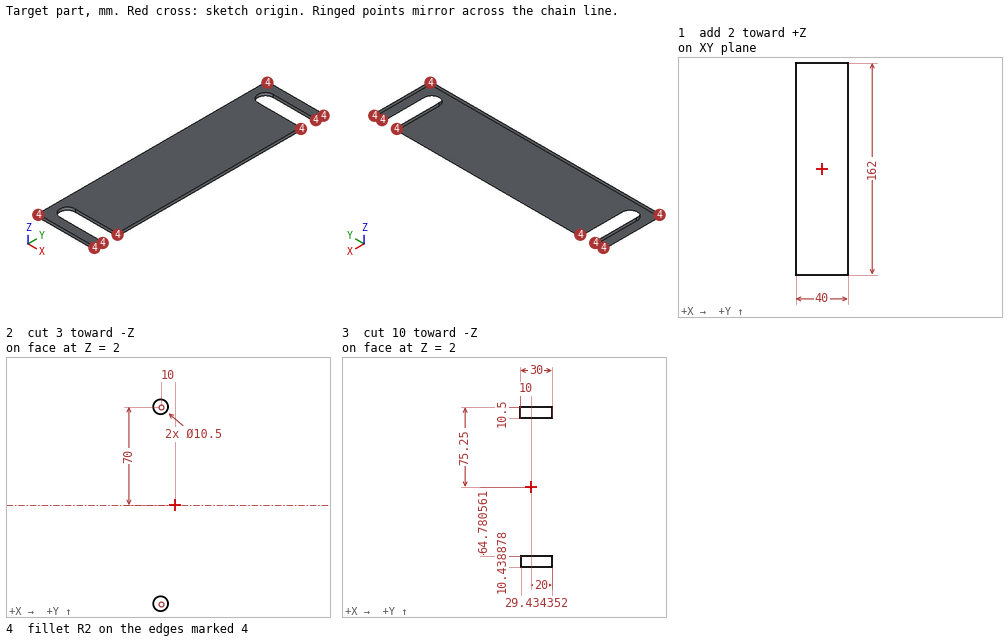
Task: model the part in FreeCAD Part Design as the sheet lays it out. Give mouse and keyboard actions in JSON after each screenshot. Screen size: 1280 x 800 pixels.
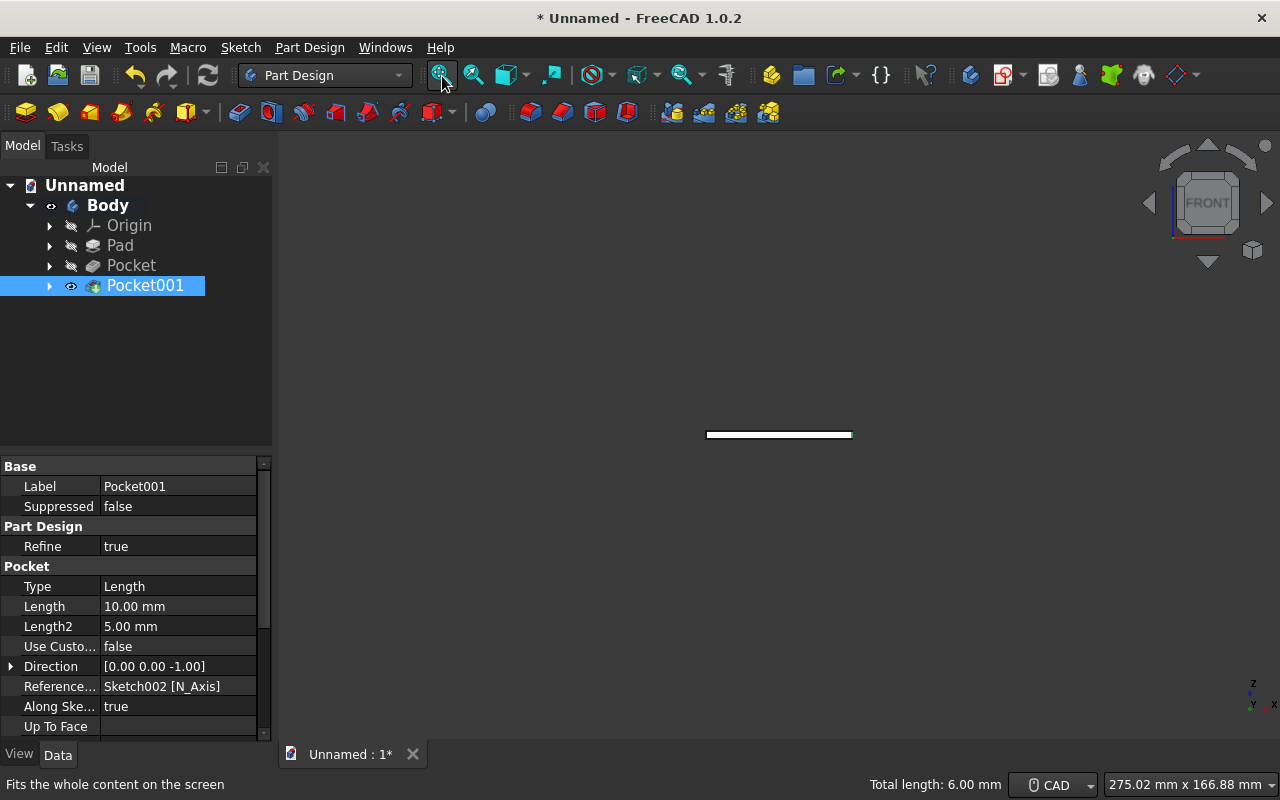
{"action": "left_click", "coordinate": [442, 76]}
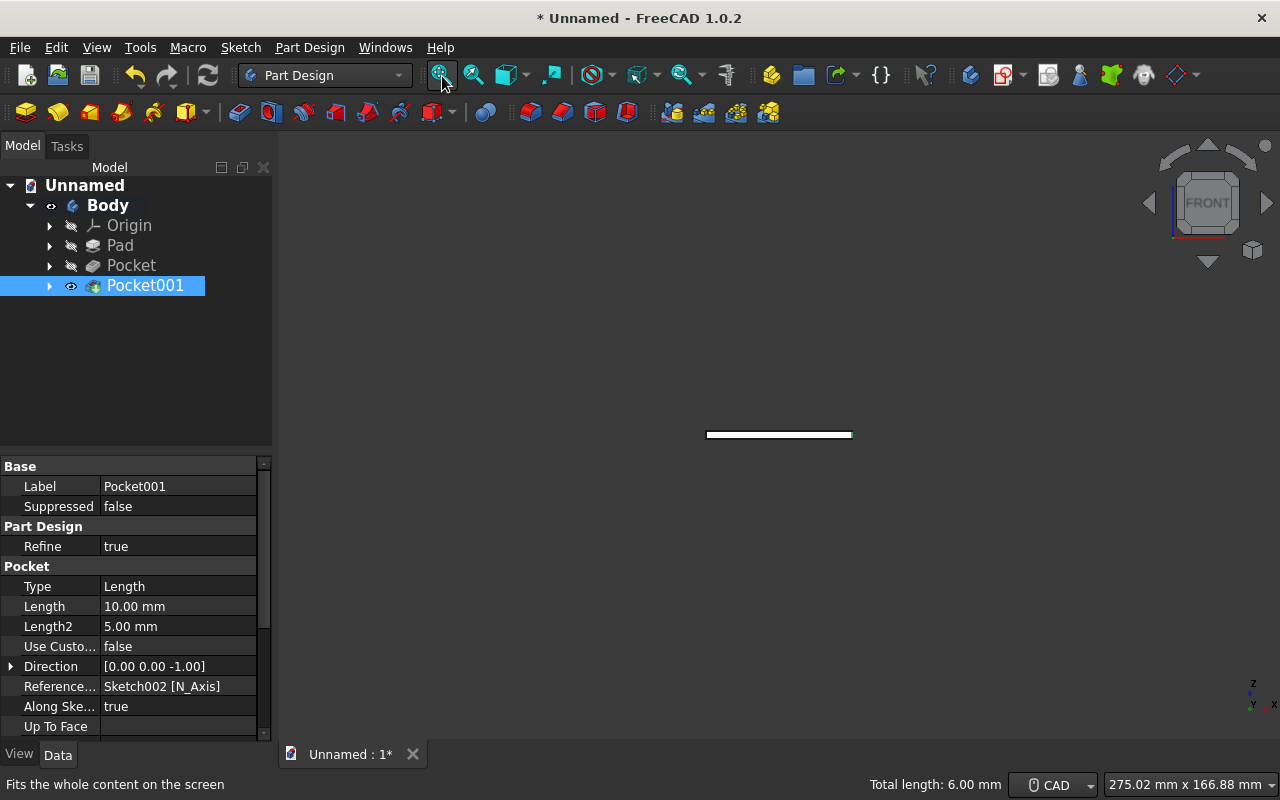
{"action": "scroll", "coordinate": [852, 434], "scroll_direction": "up", "scroll_amount": 9}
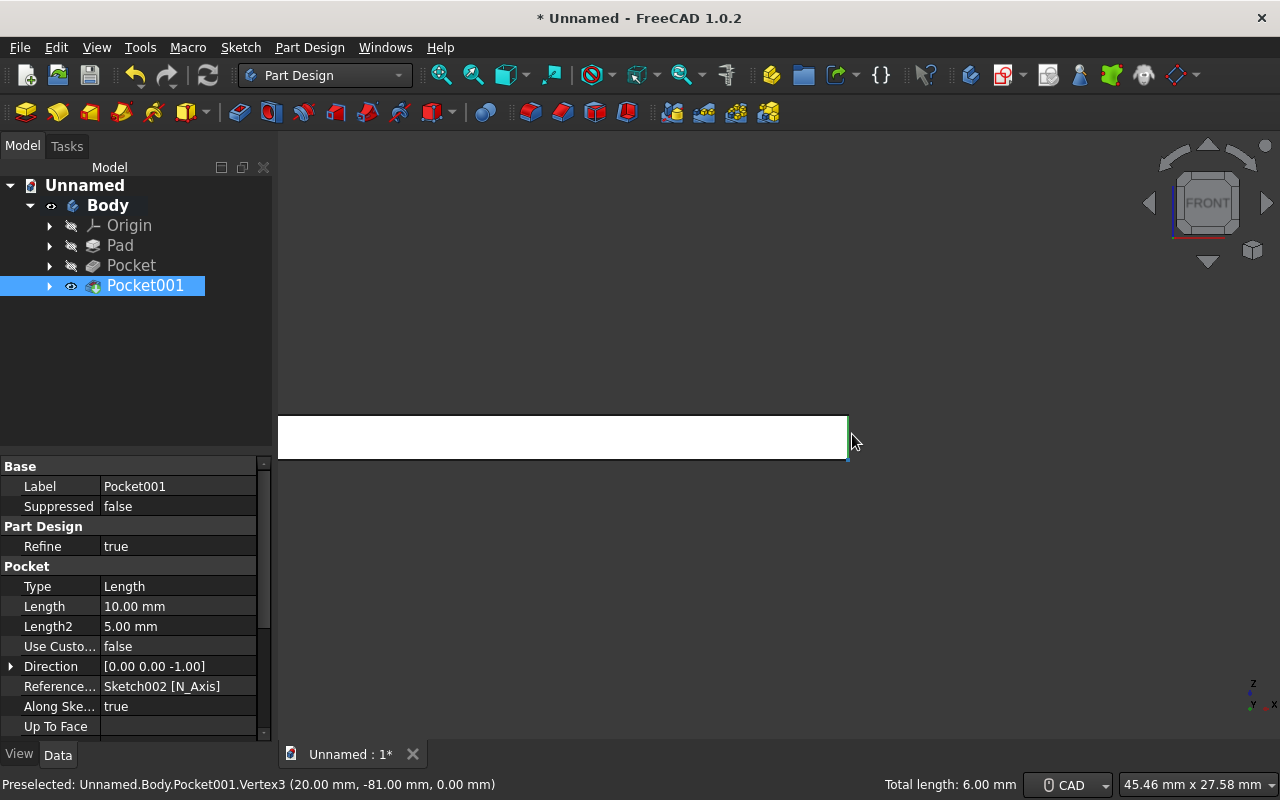
{"action": "left_click", "coordinate": [442, 76]}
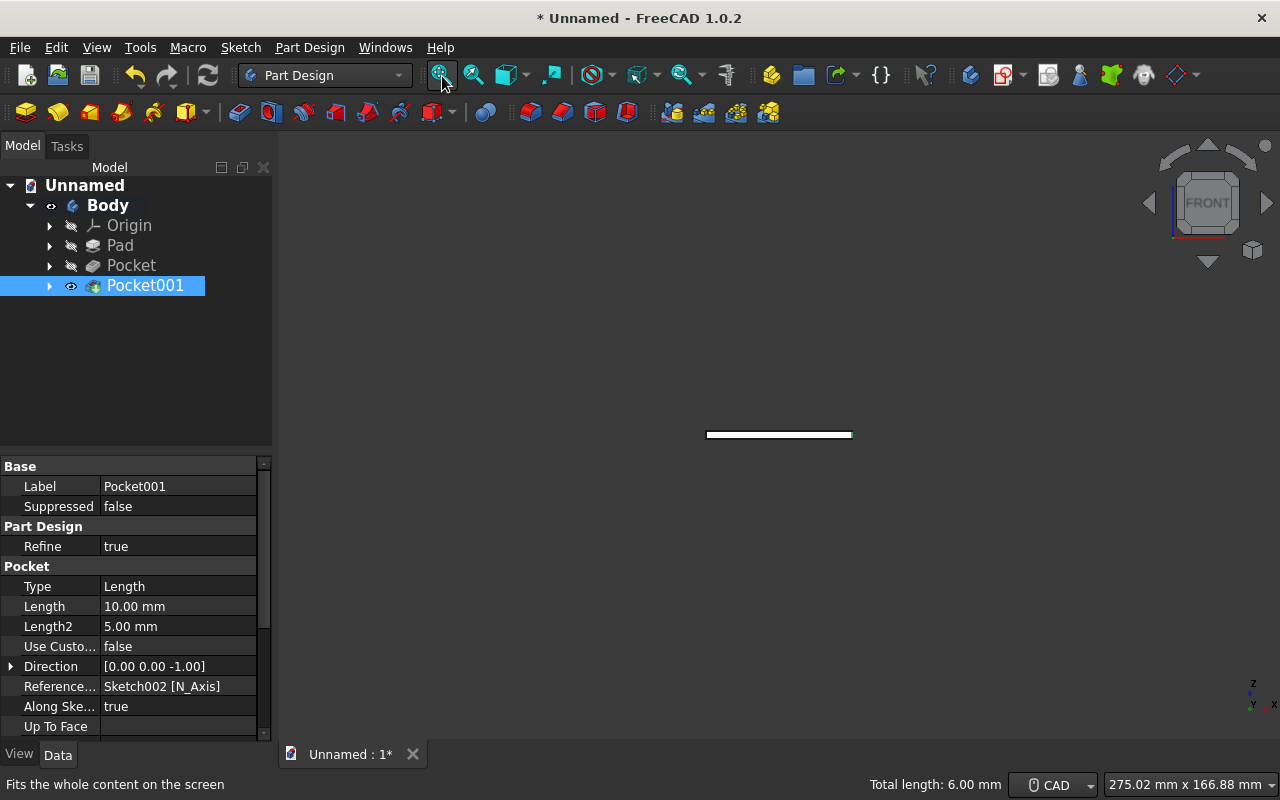
{"action": "key", "text": "3"}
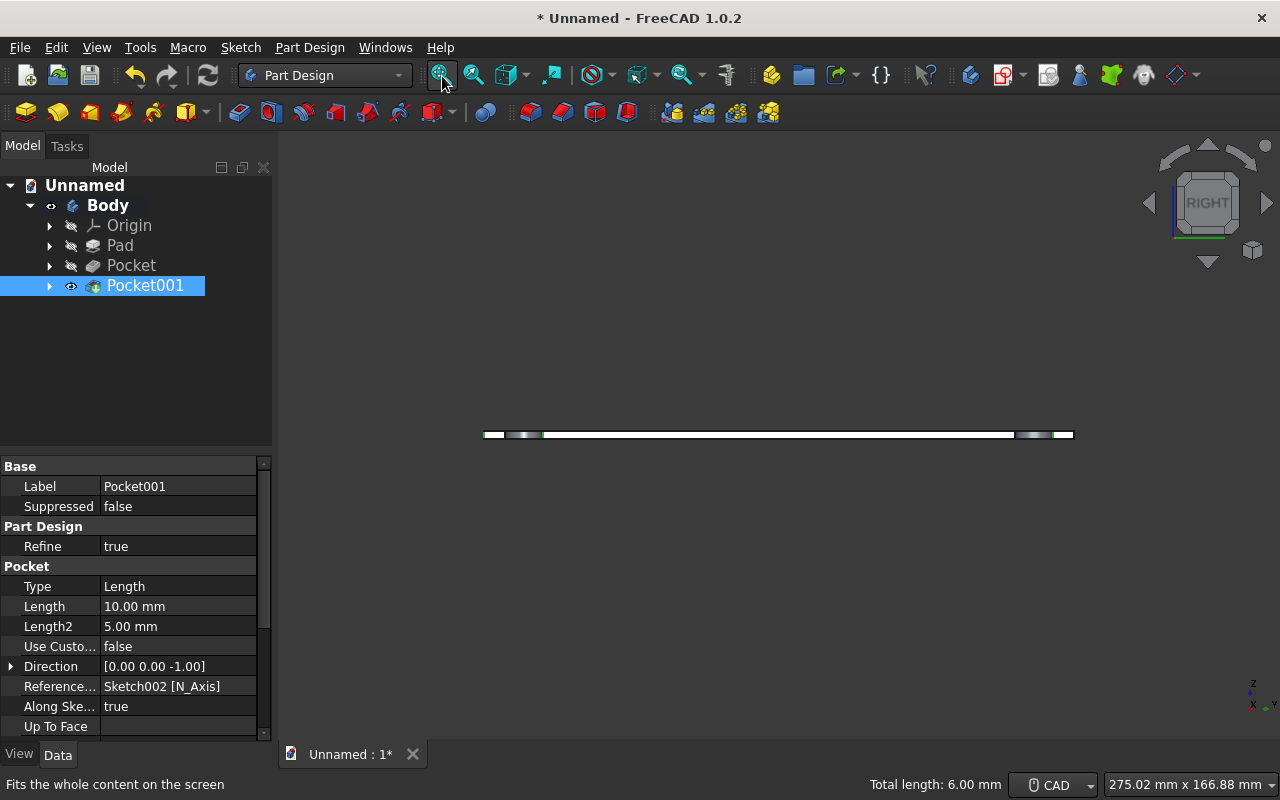
{"action": "scroll", "coordinate": [1015, 434], "scroll_direction": "up", "scroll_amount": 9}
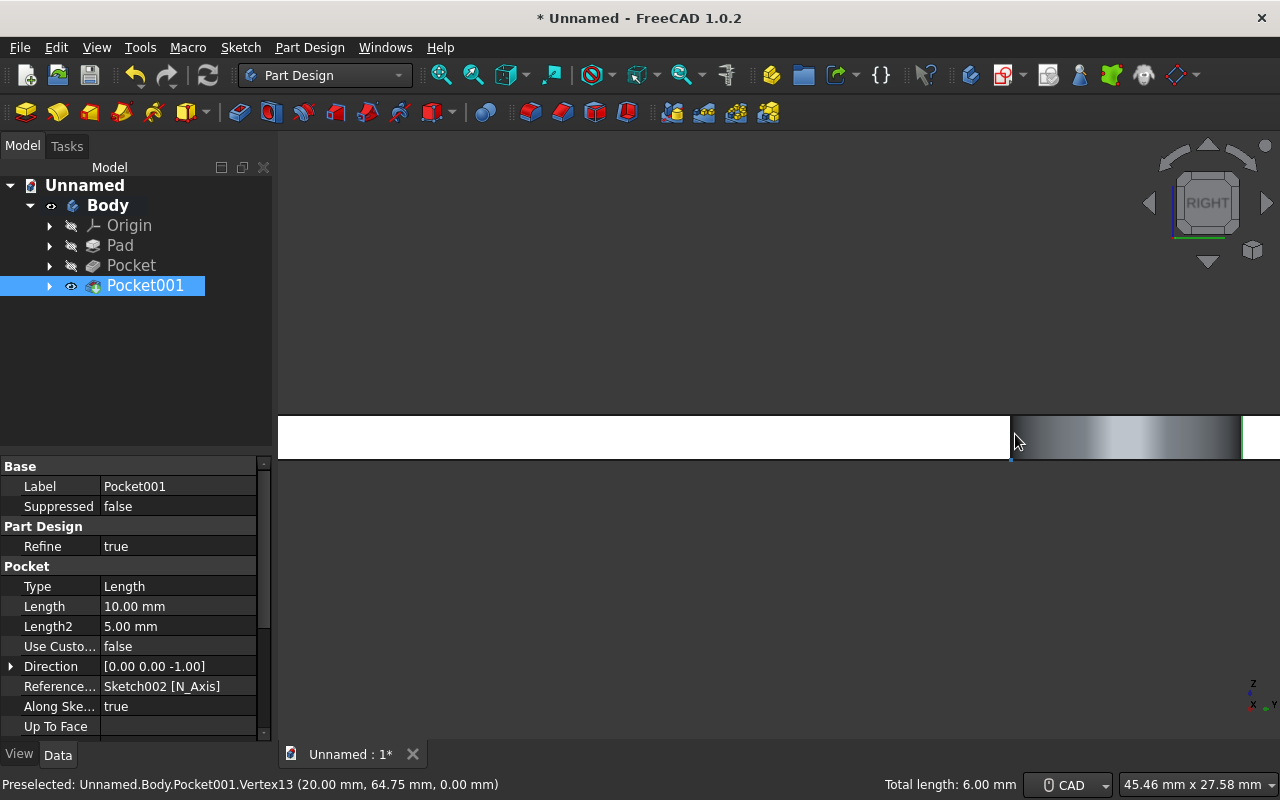
{"action": "left_click", "coordinate": [1011, 437], "text": "ctrl"}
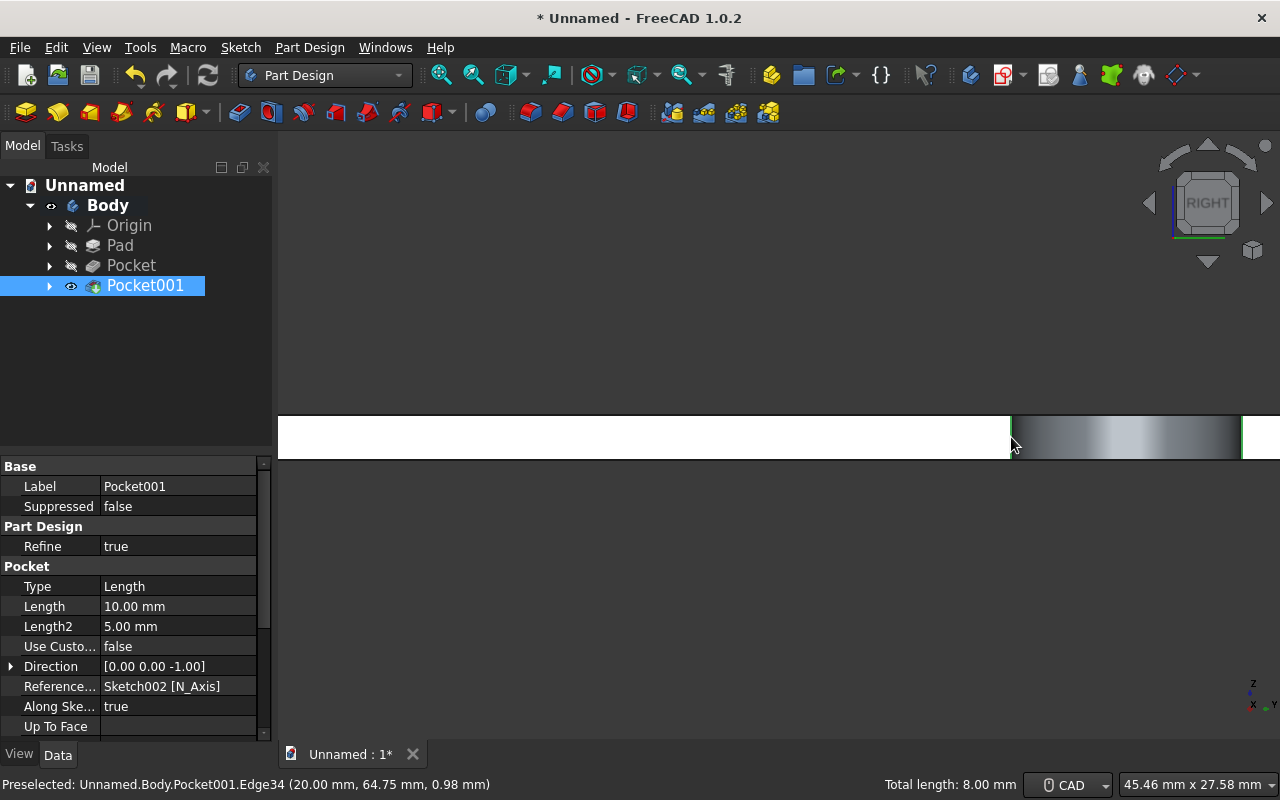
{"action": "key", "text": "v f"}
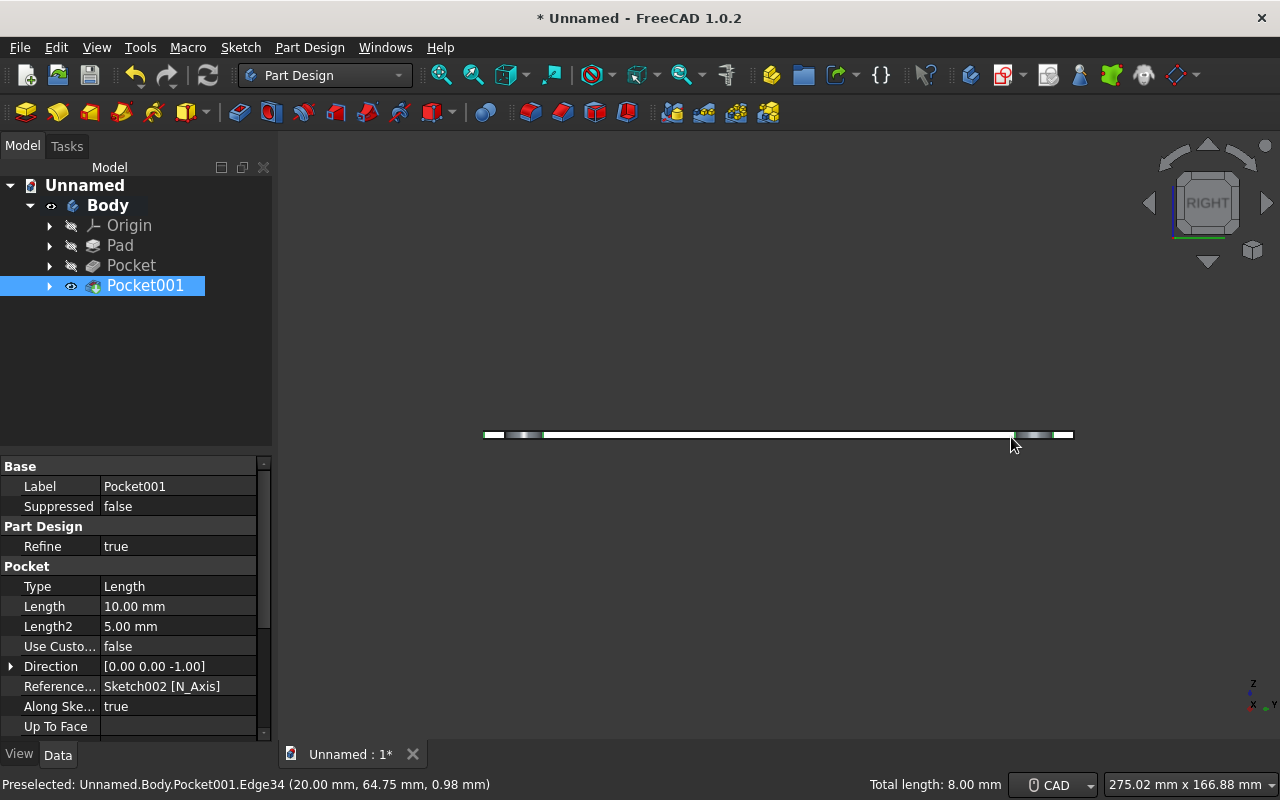
{"action": "key", "text": "5"}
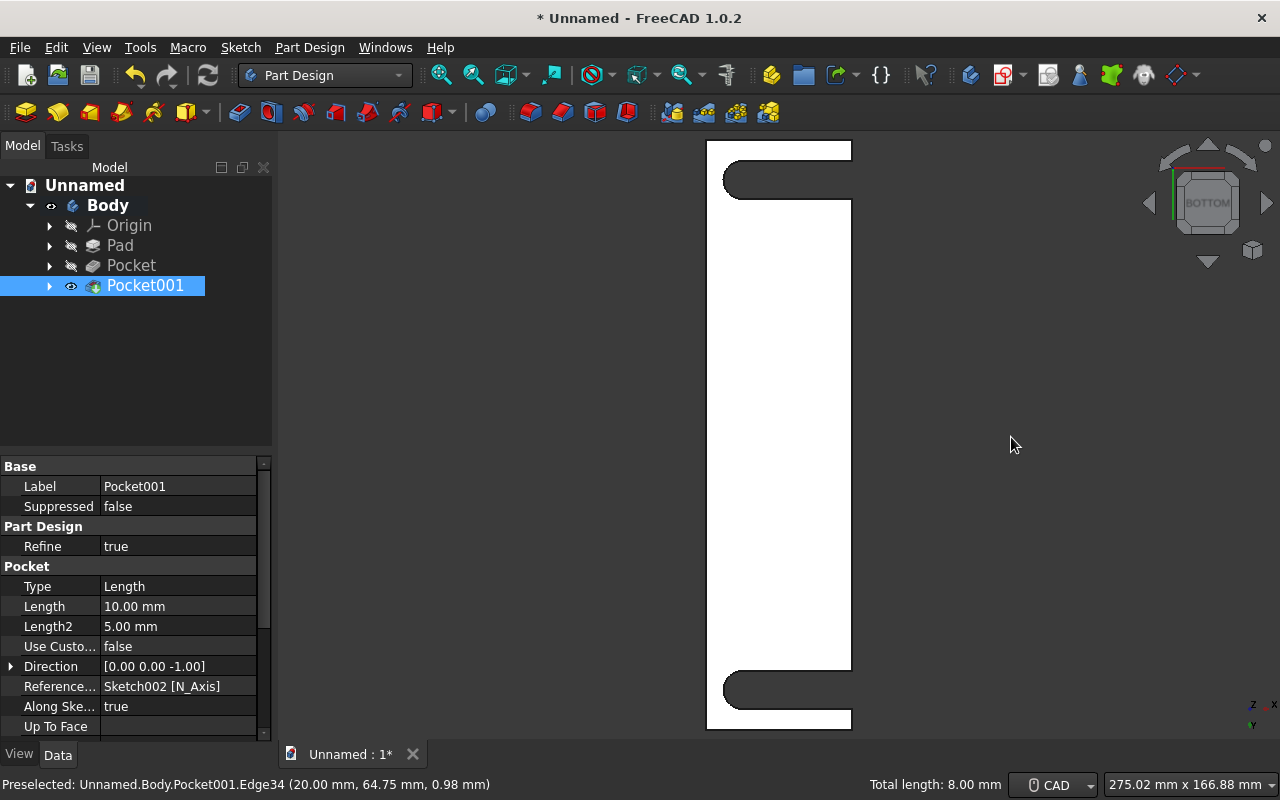
{"action": "scroll", "coordinate": [852, 160], "scroll_direction": "up", "scroll_amount": 9}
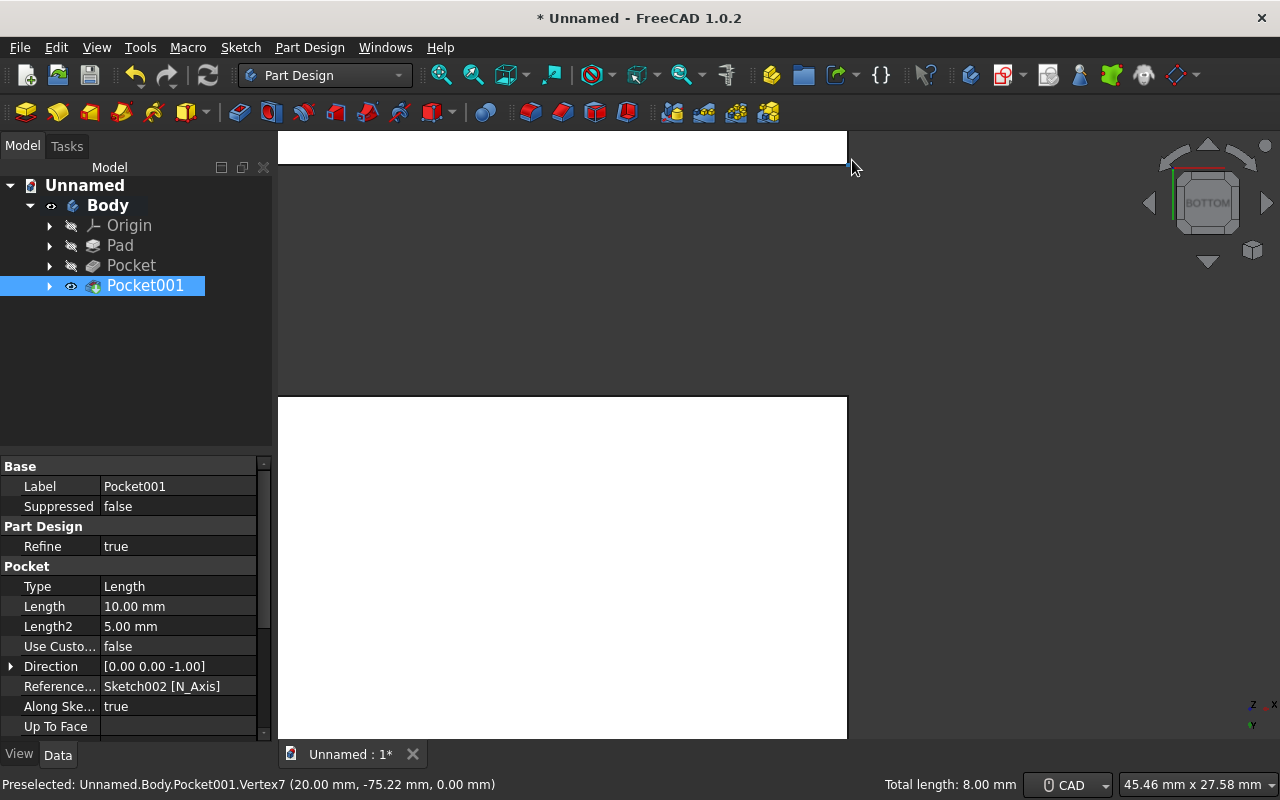
{"action": "left_click", "coordinate": [442, 76]}